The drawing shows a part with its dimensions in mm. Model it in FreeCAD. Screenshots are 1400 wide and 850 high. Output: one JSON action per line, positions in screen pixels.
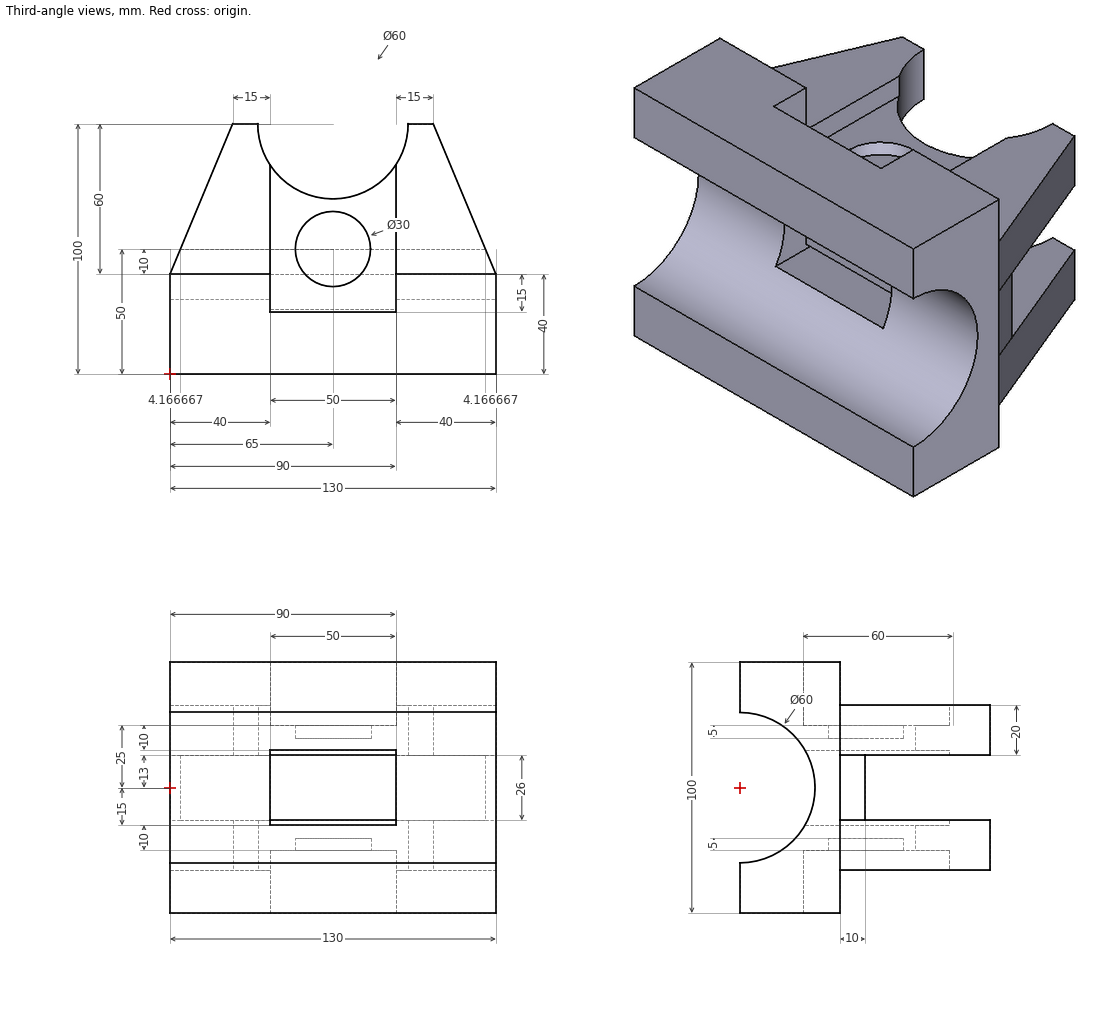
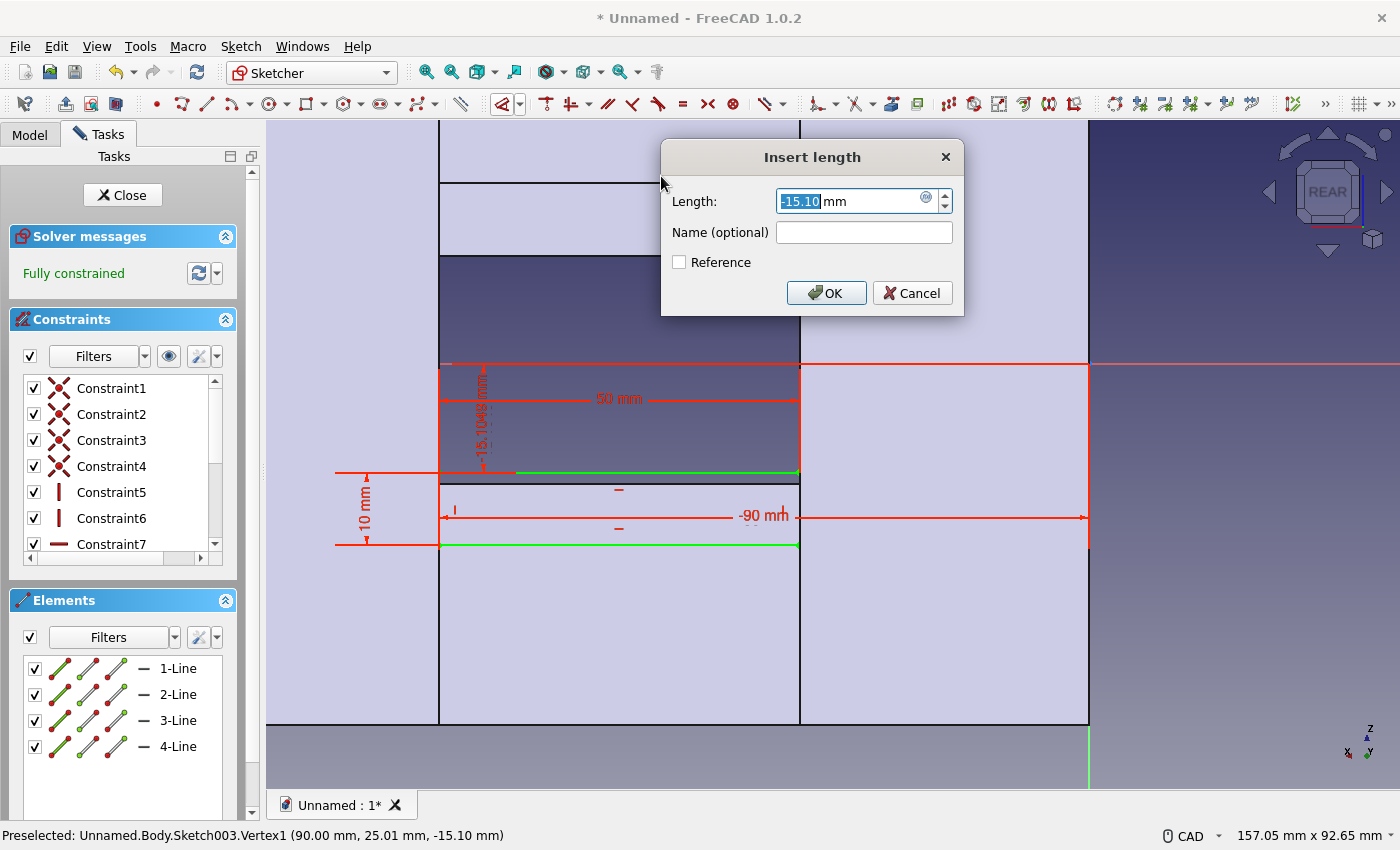
{"action": "type", "text": "-15"}
{"action": "key", "text": "Return"}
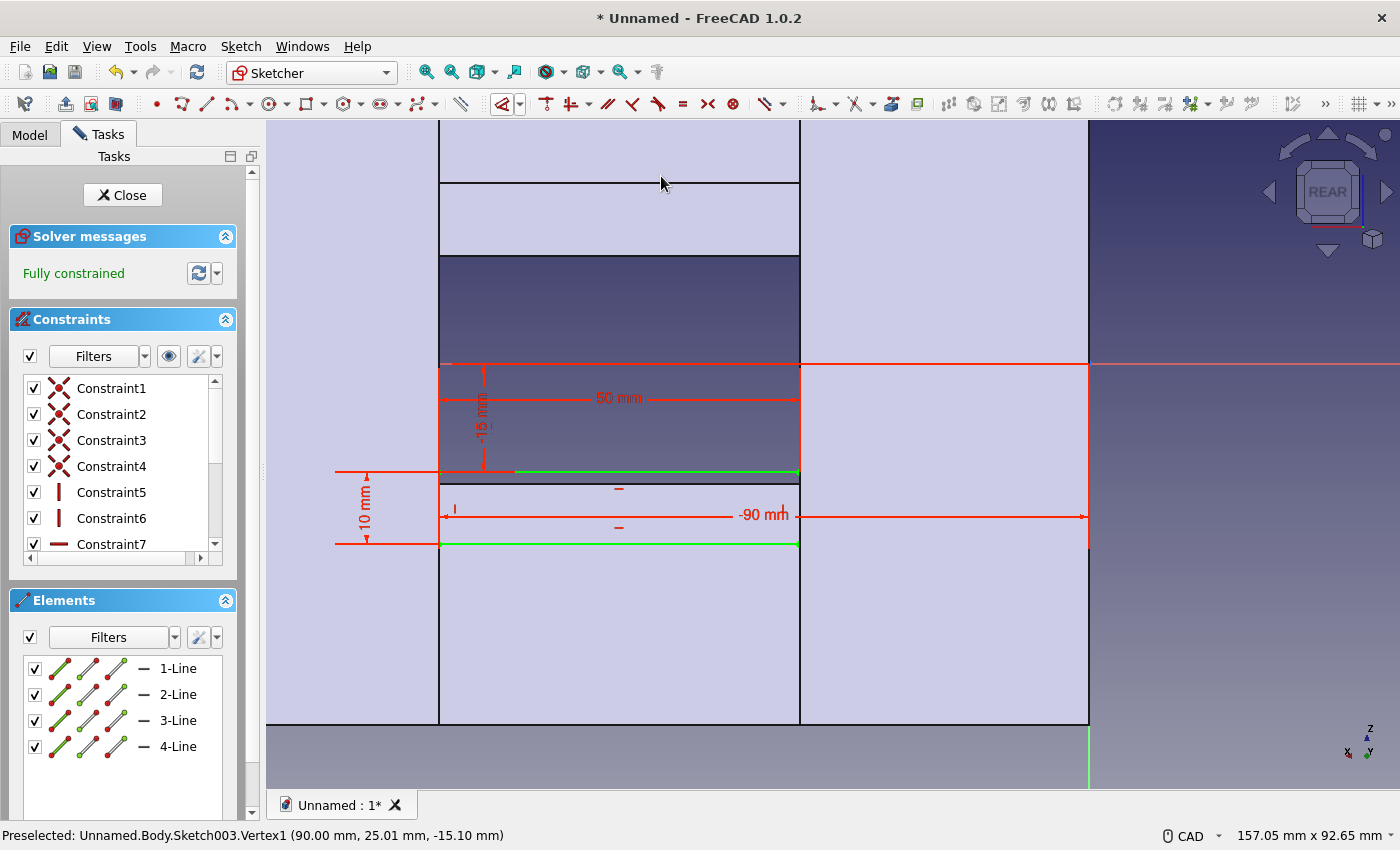
{"action": "left_click", "coordinate": [123, 195]}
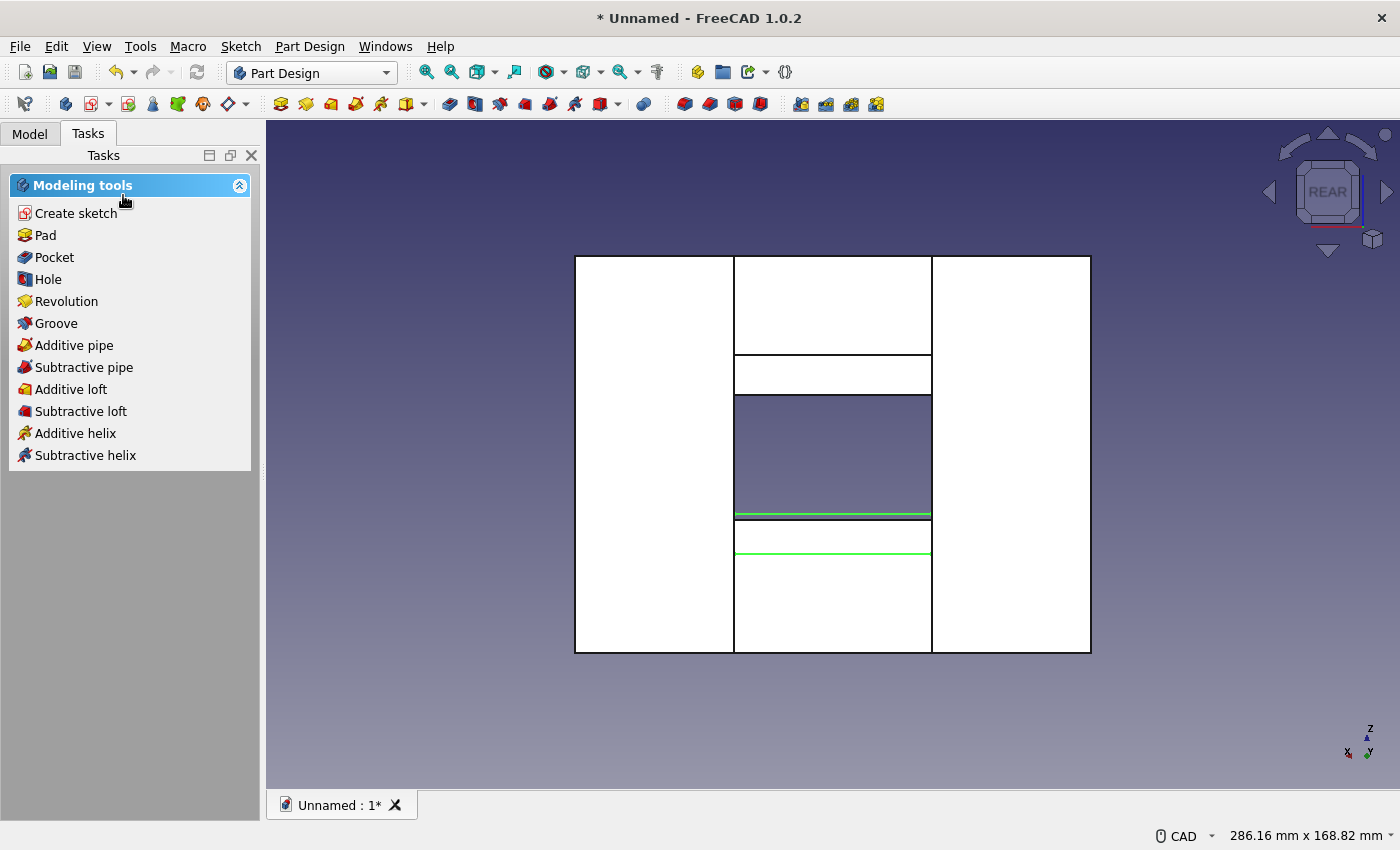
{"action": "left_click", "coordinate": [281, 104]}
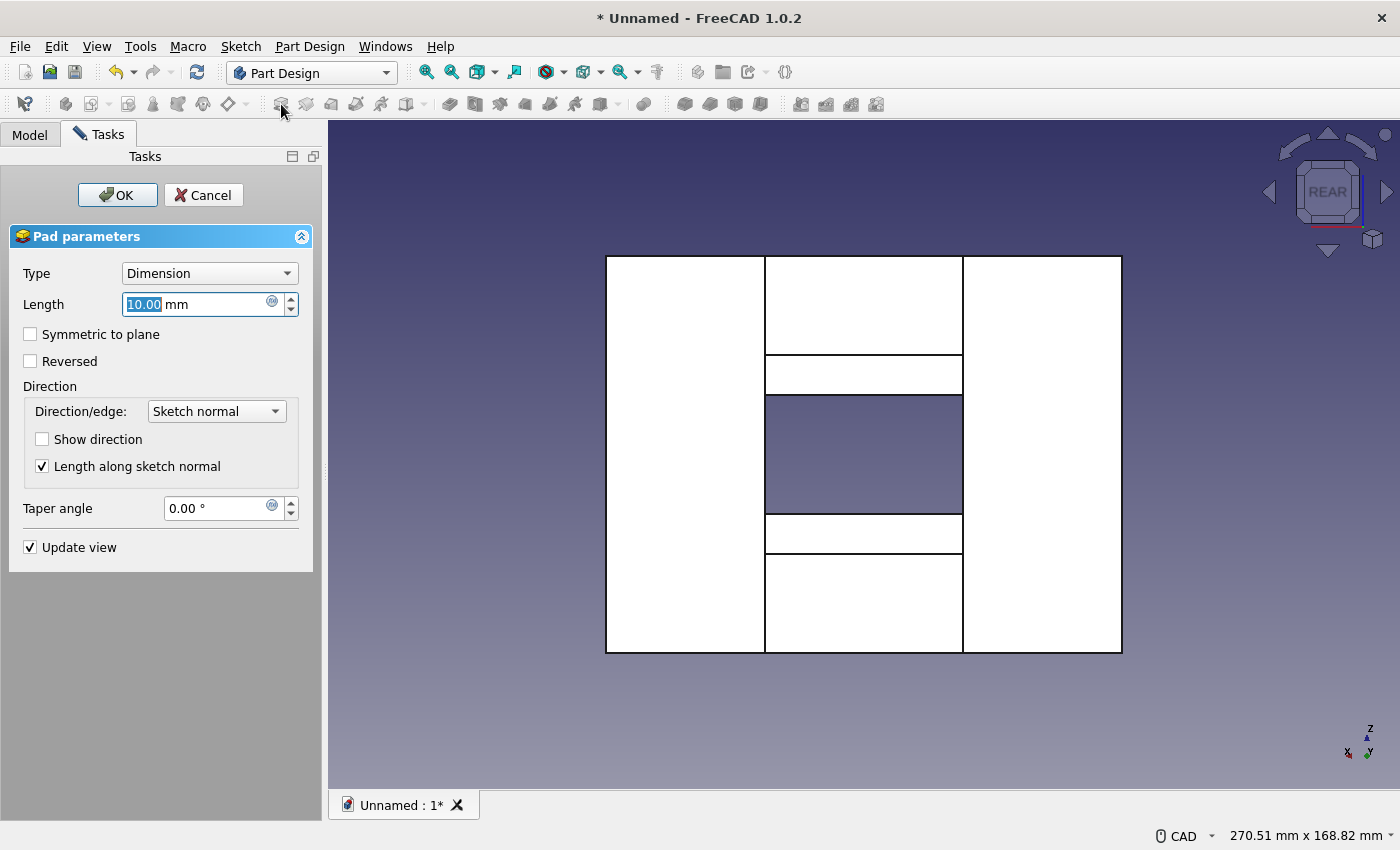
{"action": "type", "text": "60"}
{"action": "key", "text": "Tab"}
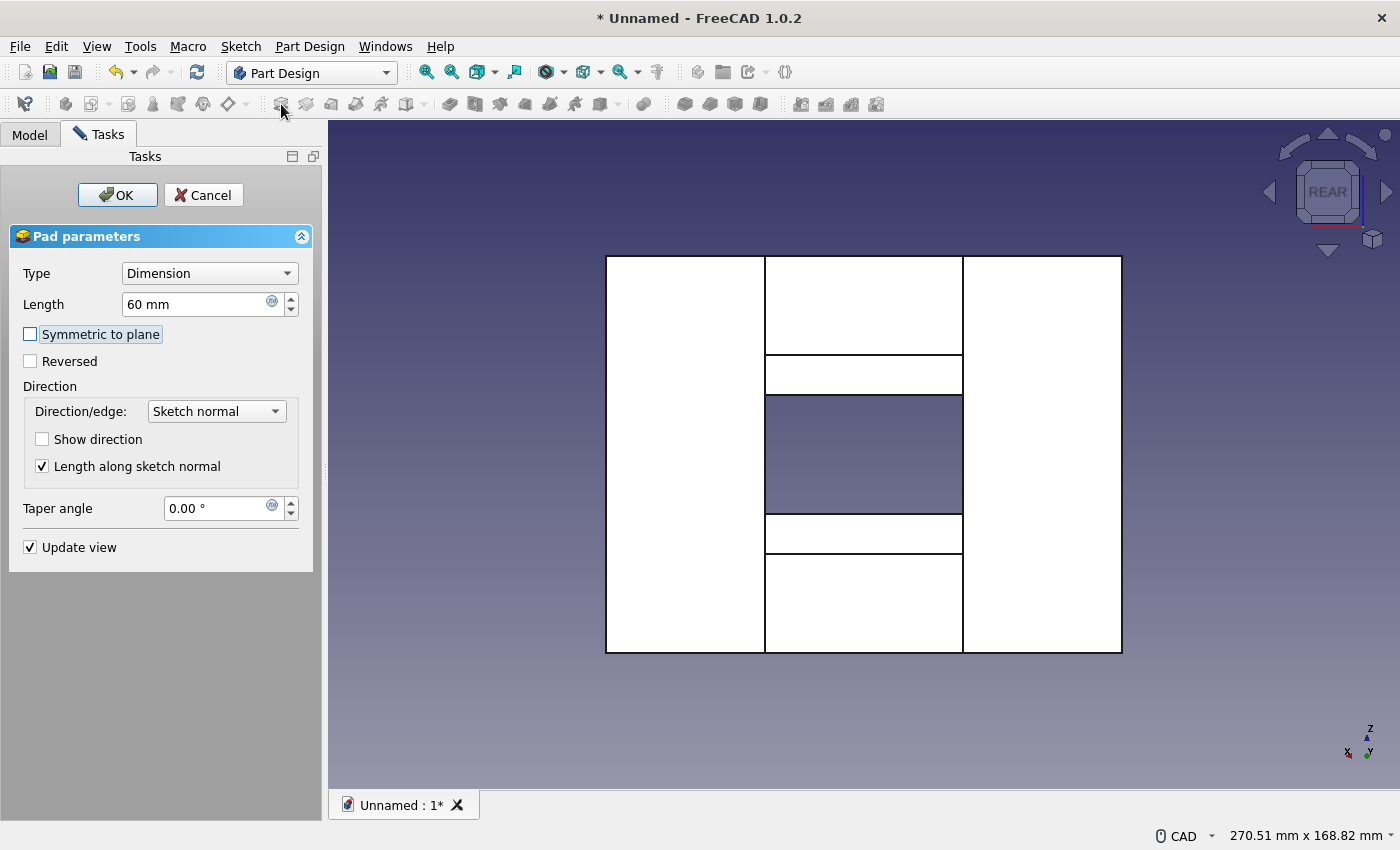
{"action": "left_click", "coordinate": [118, 195]}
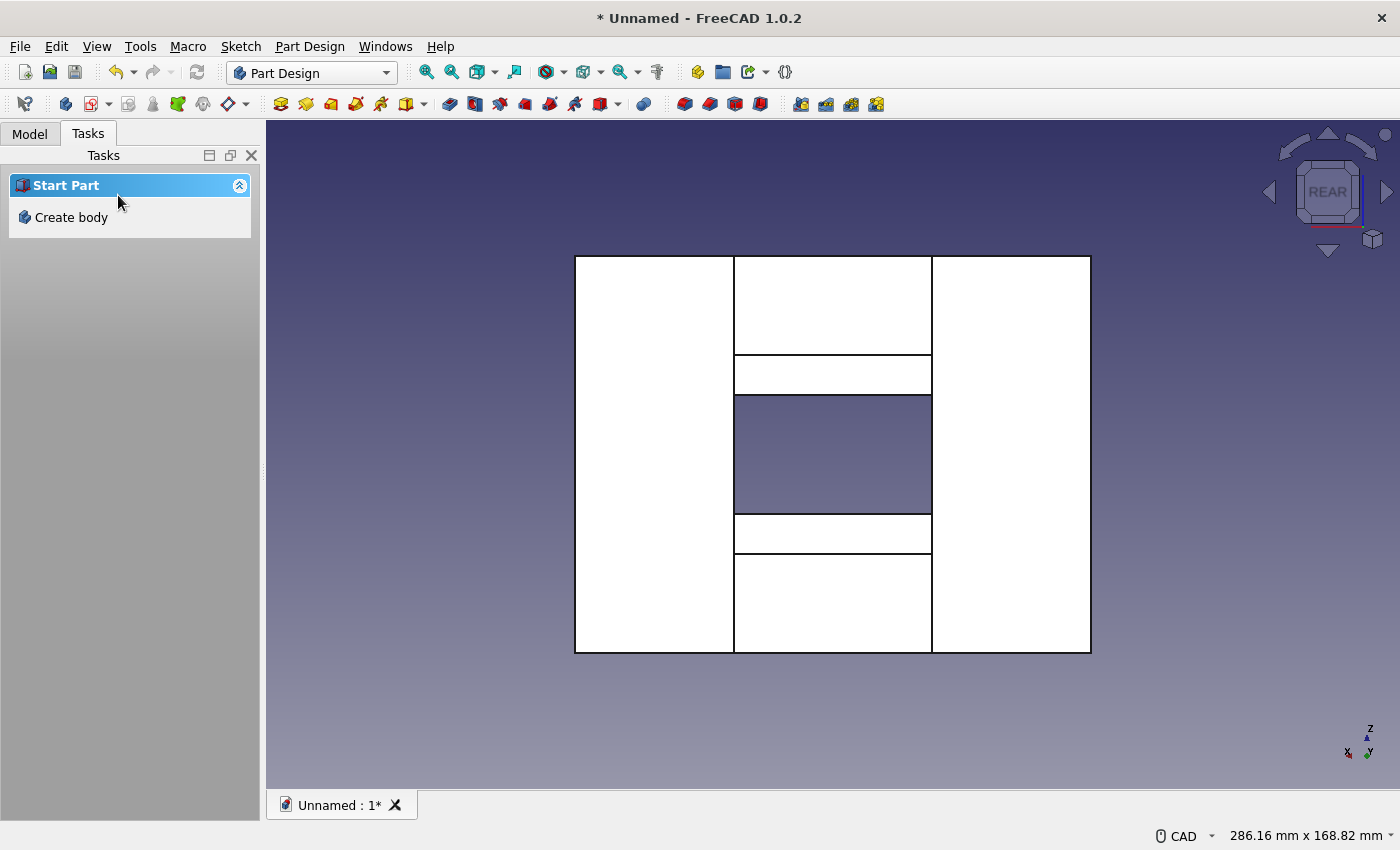
{"action": "key", "text": "0"}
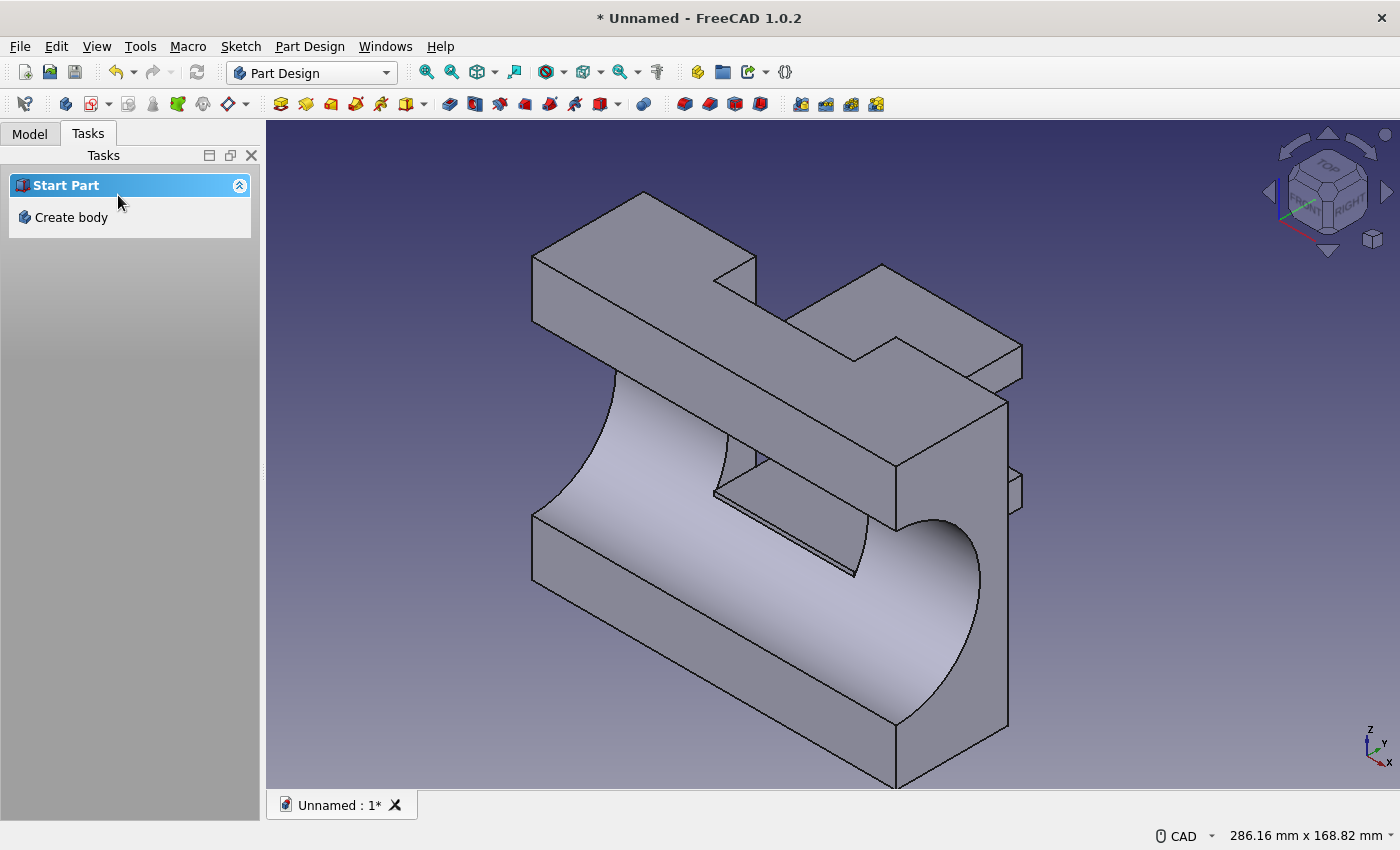
{"action": "left_click", "coordinate": [427, 72]}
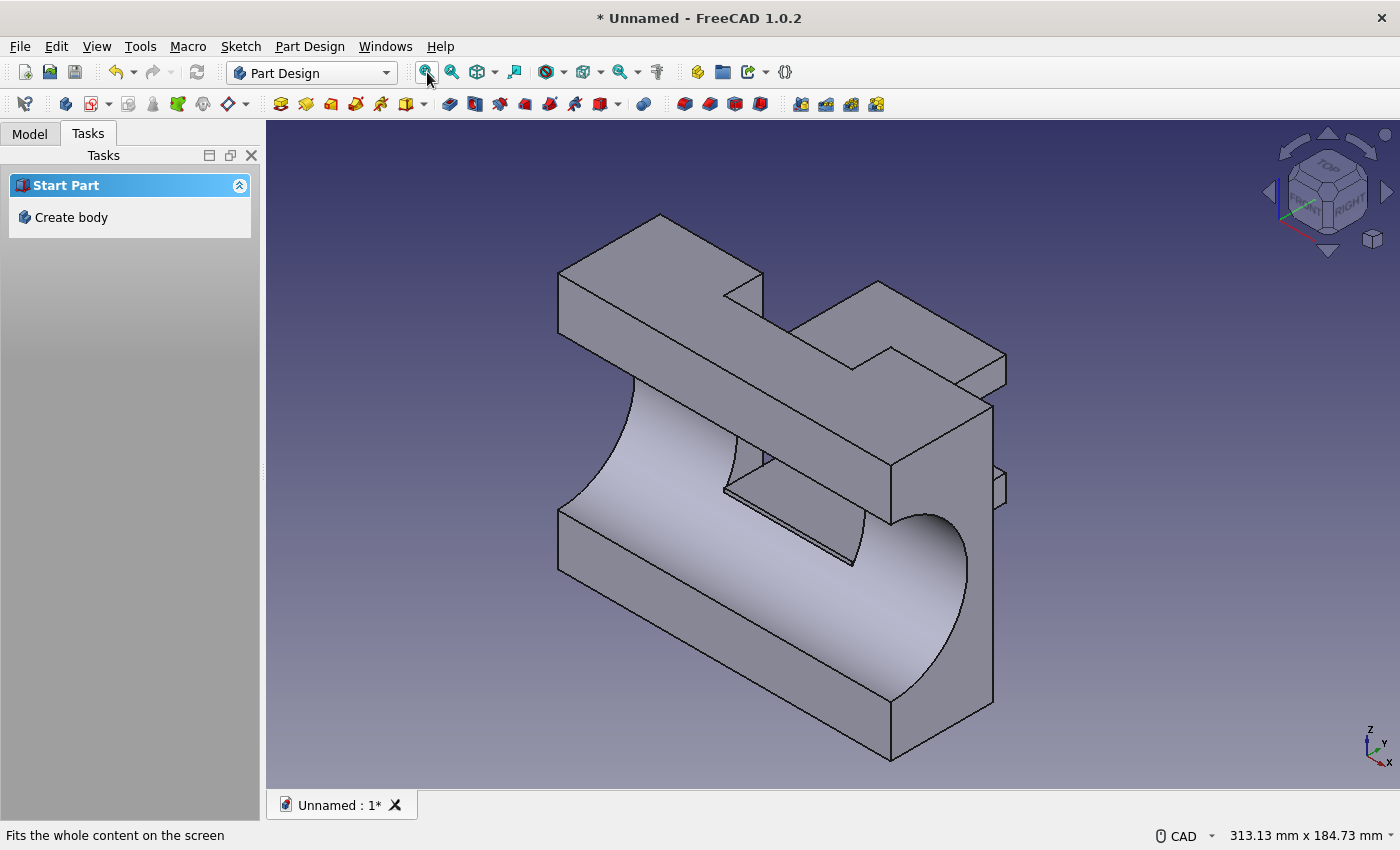
{"action": "left_click", "coordinate": [869, 338]}